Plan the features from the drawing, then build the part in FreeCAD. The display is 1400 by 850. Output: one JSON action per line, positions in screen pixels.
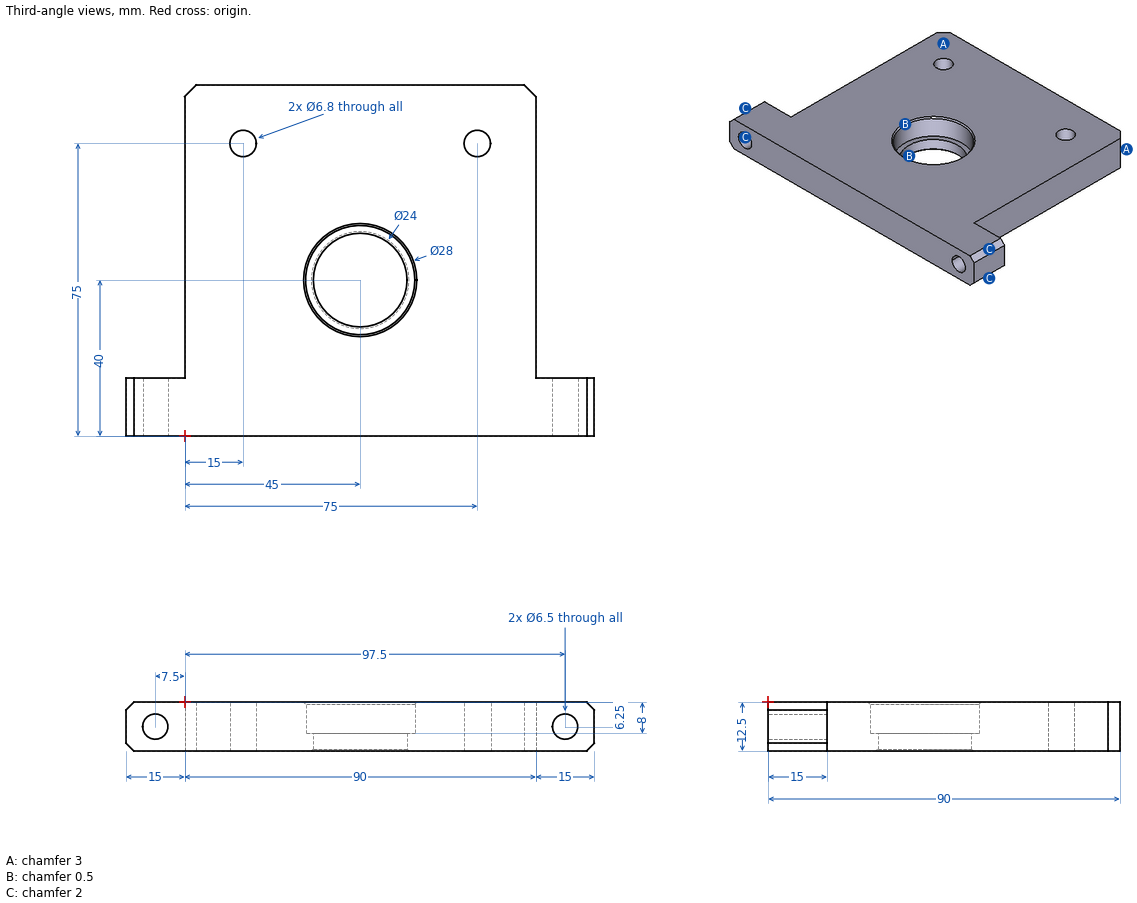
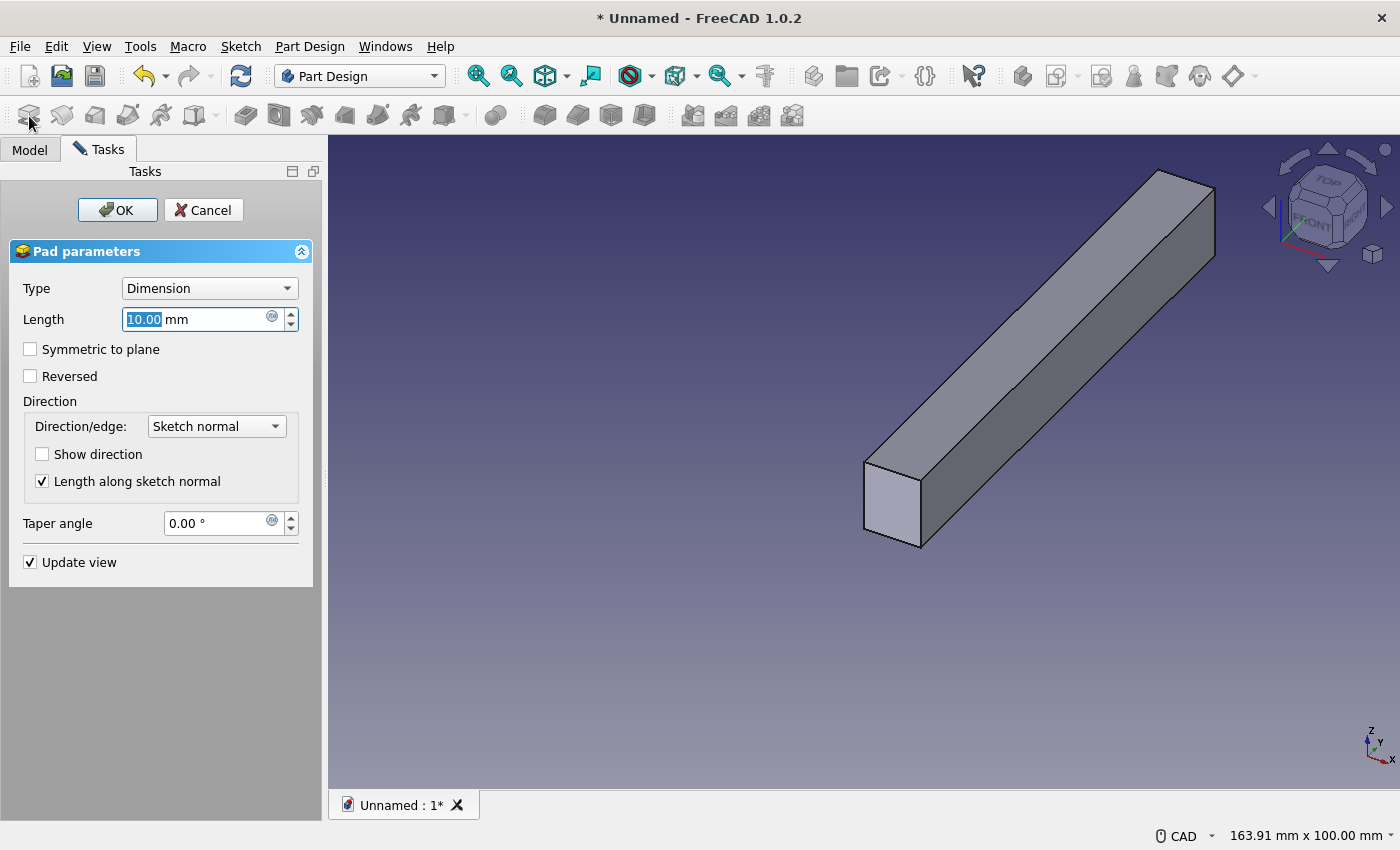
{"action": "type", "text": "90"}
{"action": "key", "text": "Tab"}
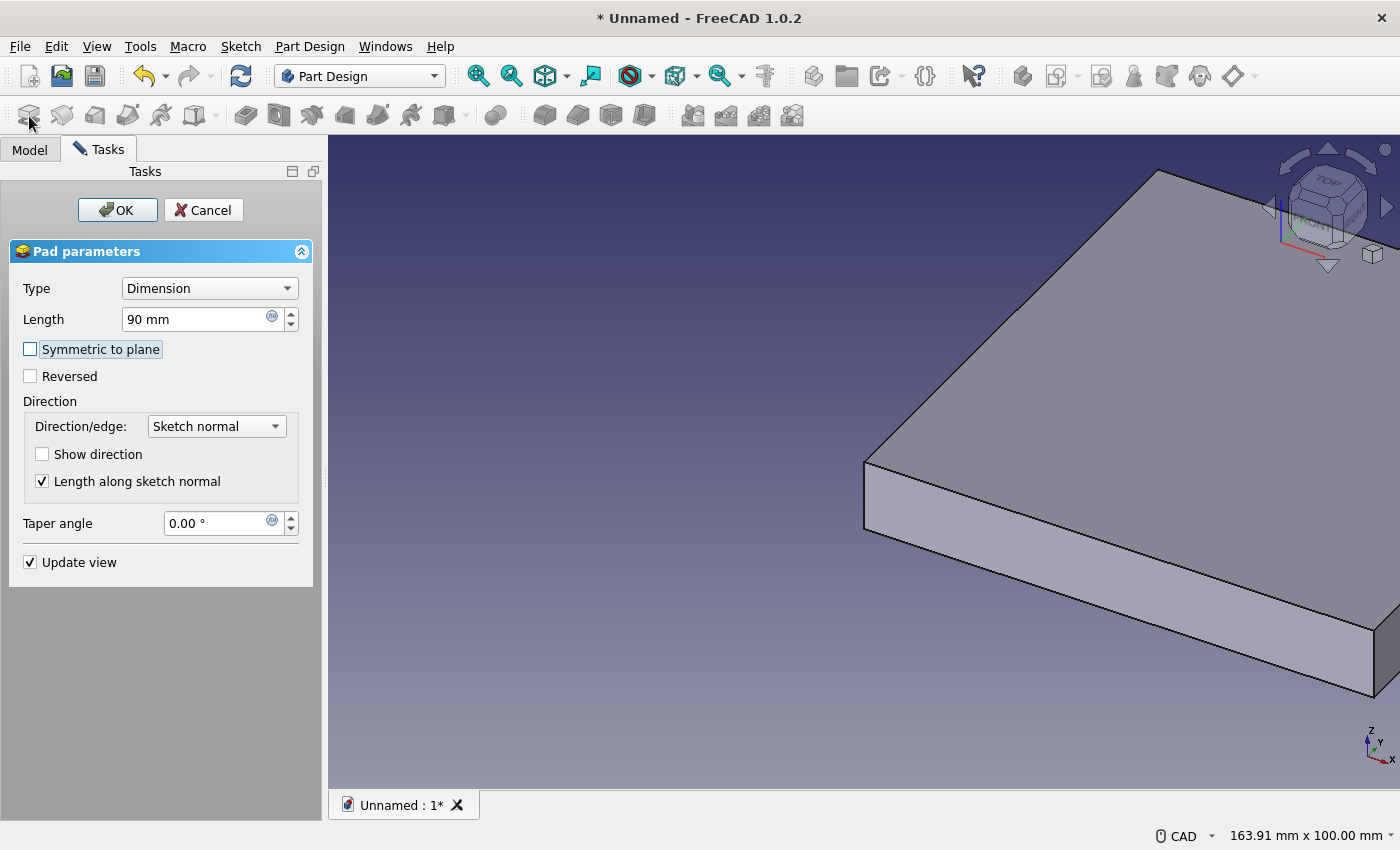
{"action": "left_click", "coordinate": [118, 210]}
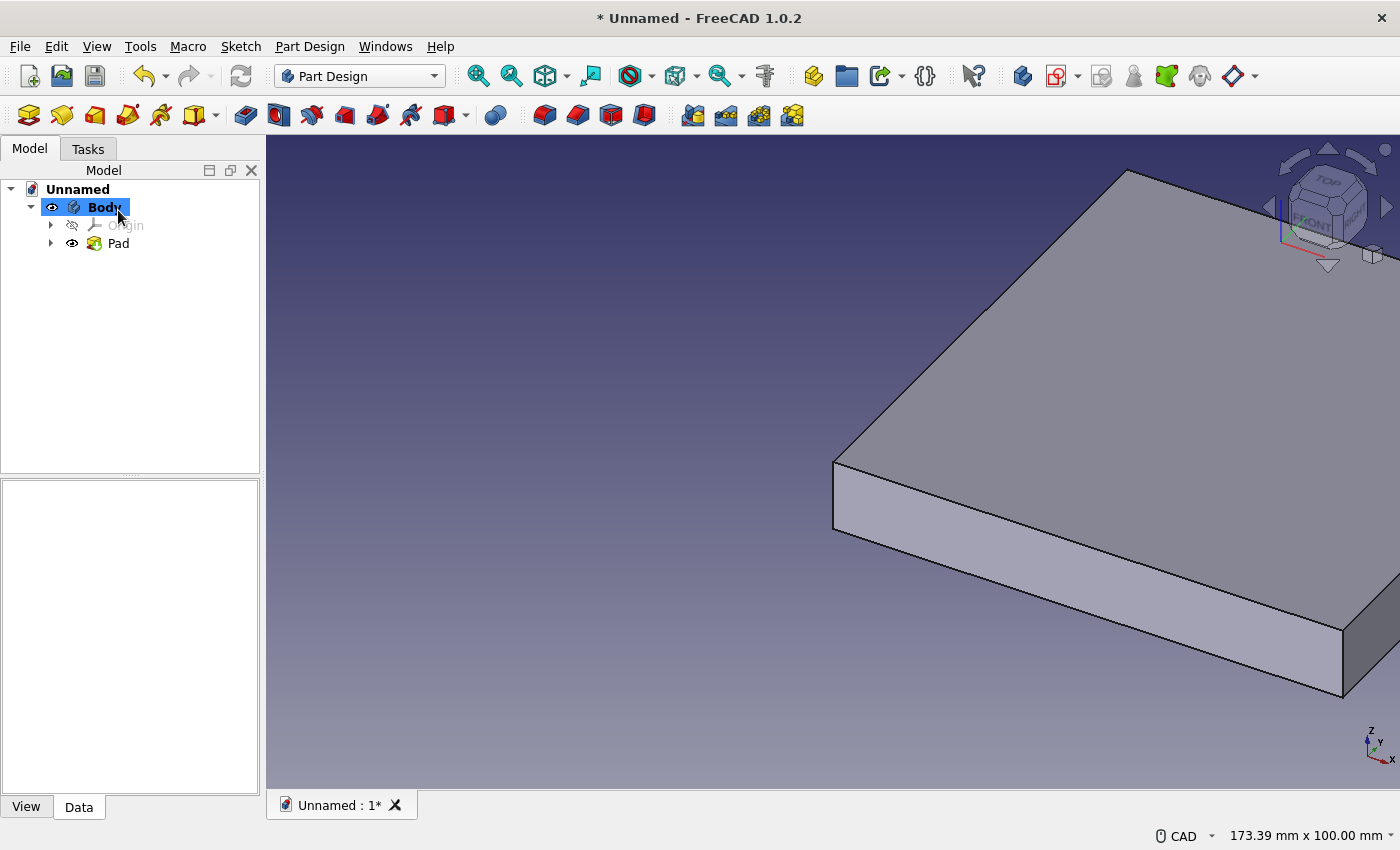
{"action": "left_click", "coordinate": [479, 76]}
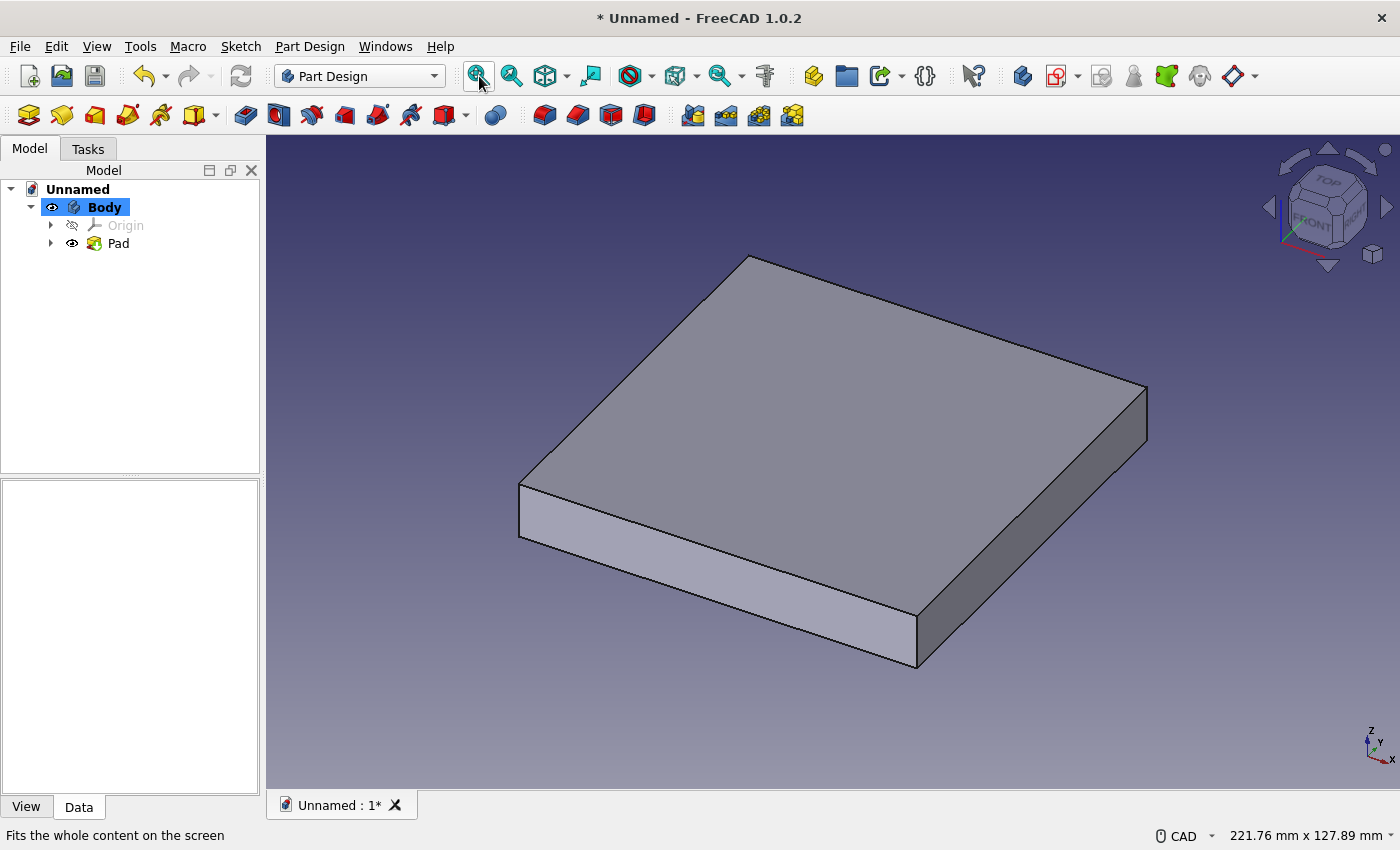
{"action": "key", "text": "0"}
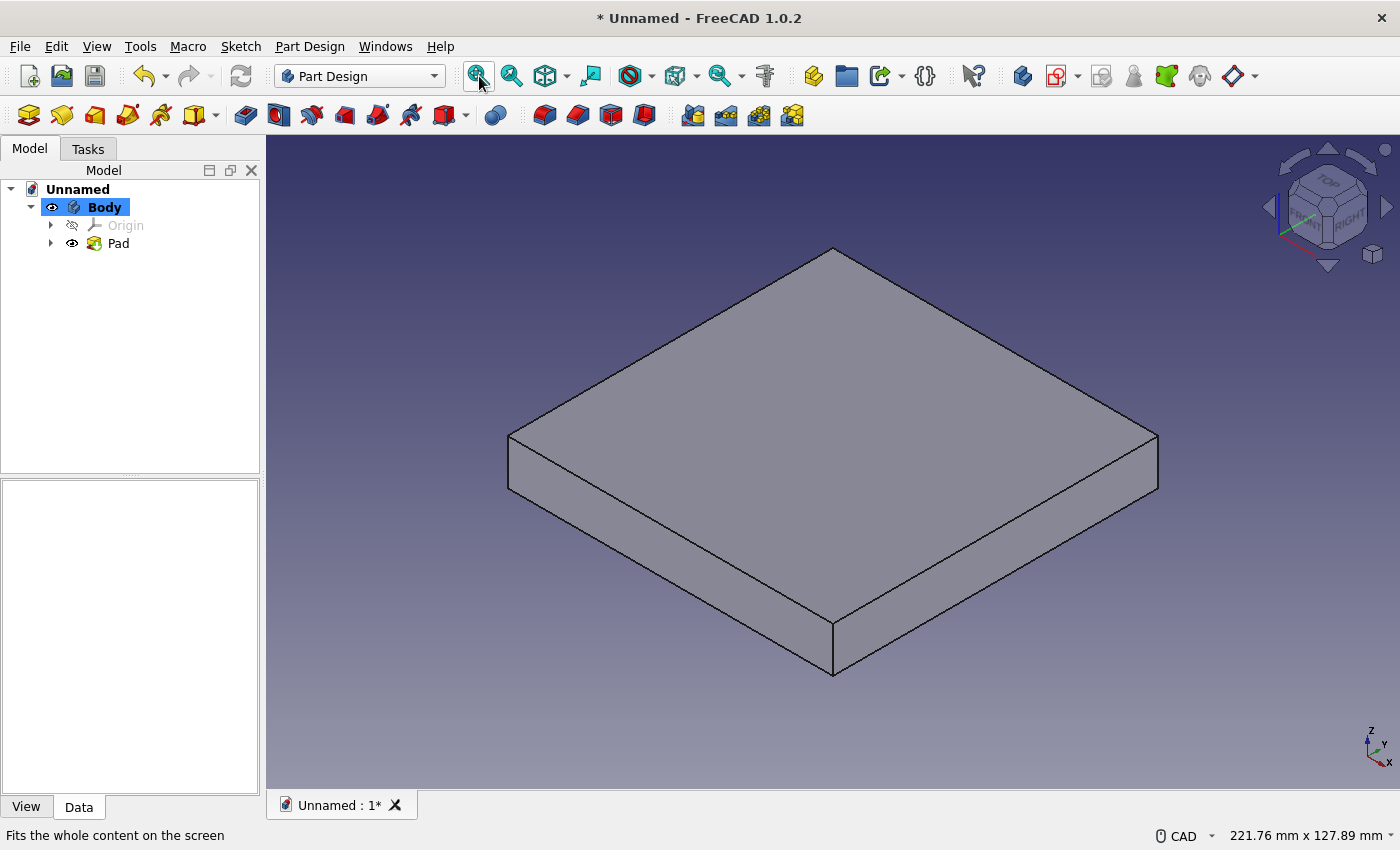
{"action": "key", "text": "2"}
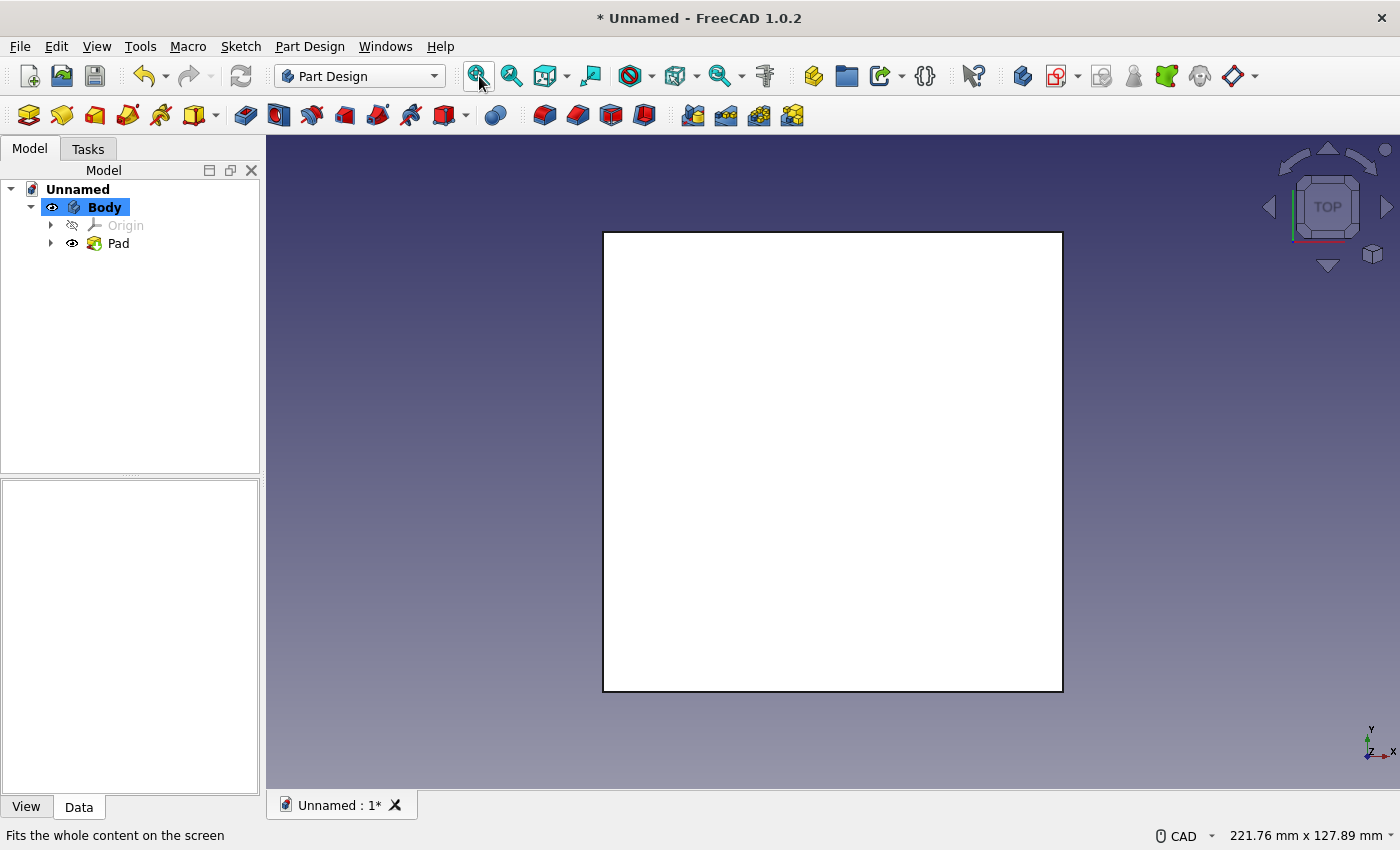
{"action": "key", "text": "1"}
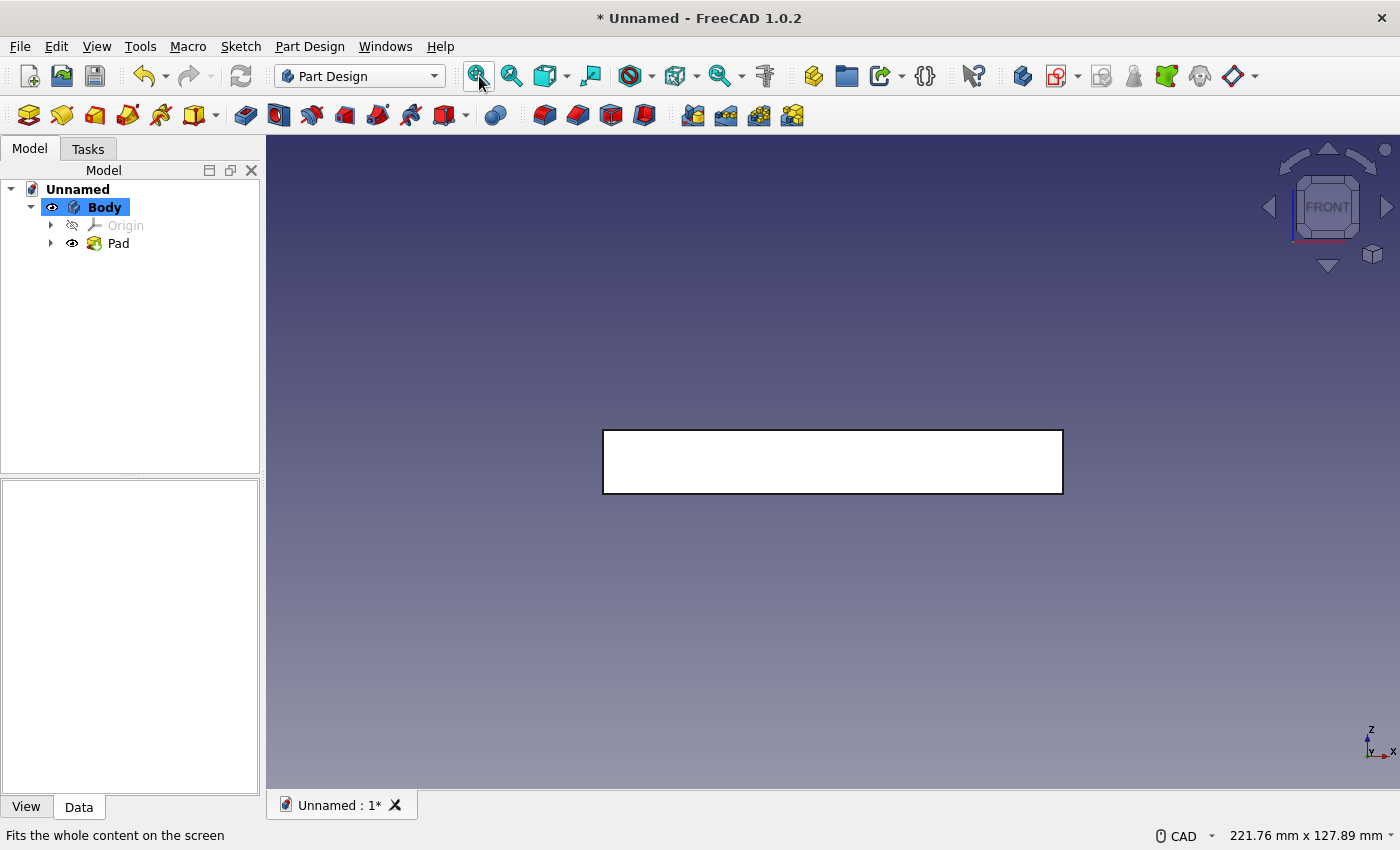
{"action": "left_click", "coordinate": [479, 76]}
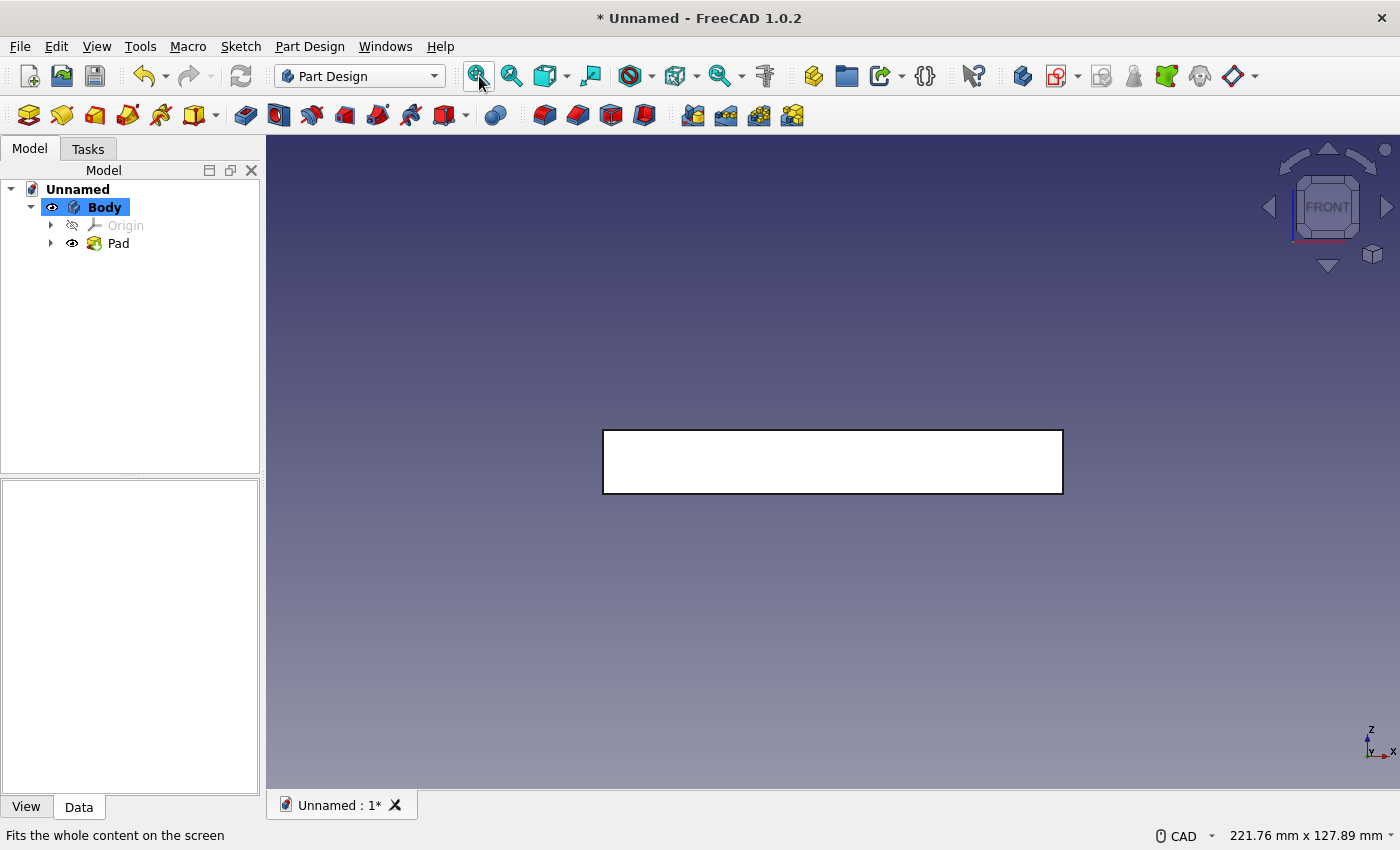
{"action": "key", "text": "3"}